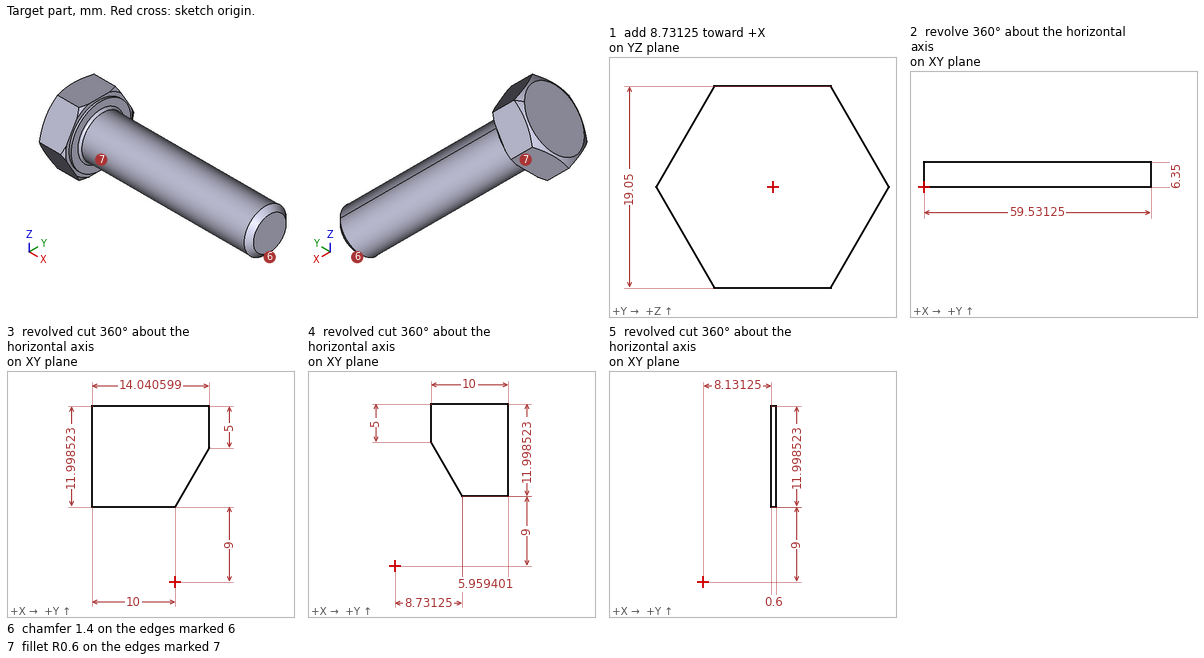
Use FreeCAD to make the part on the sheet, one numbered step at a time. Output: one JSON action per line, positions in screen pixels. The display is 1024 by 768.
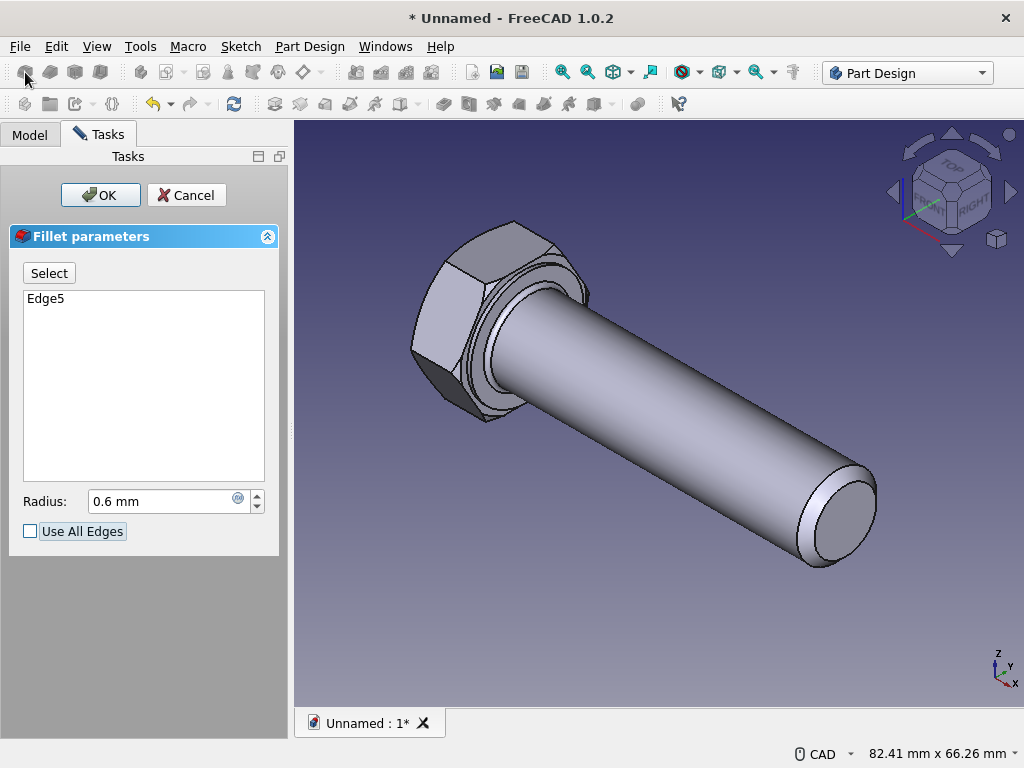
{"action": "left_click", "coordinate": [101, 195]}